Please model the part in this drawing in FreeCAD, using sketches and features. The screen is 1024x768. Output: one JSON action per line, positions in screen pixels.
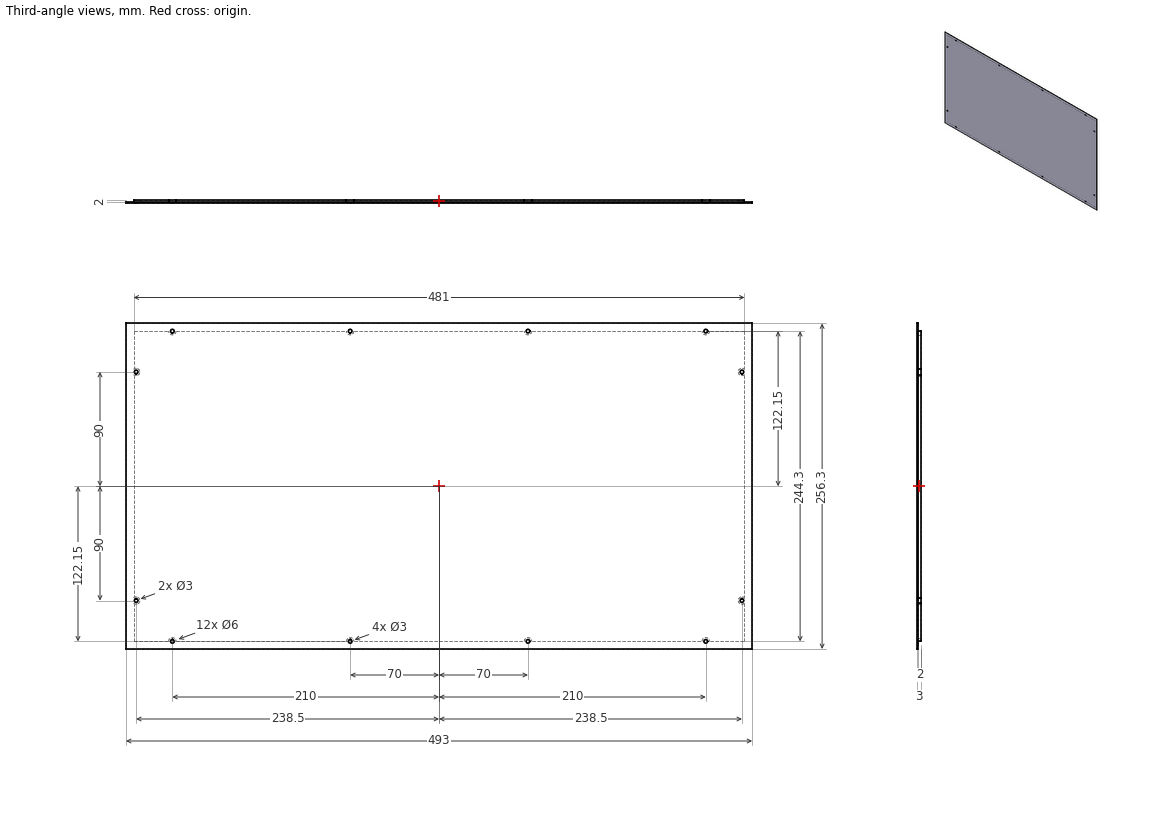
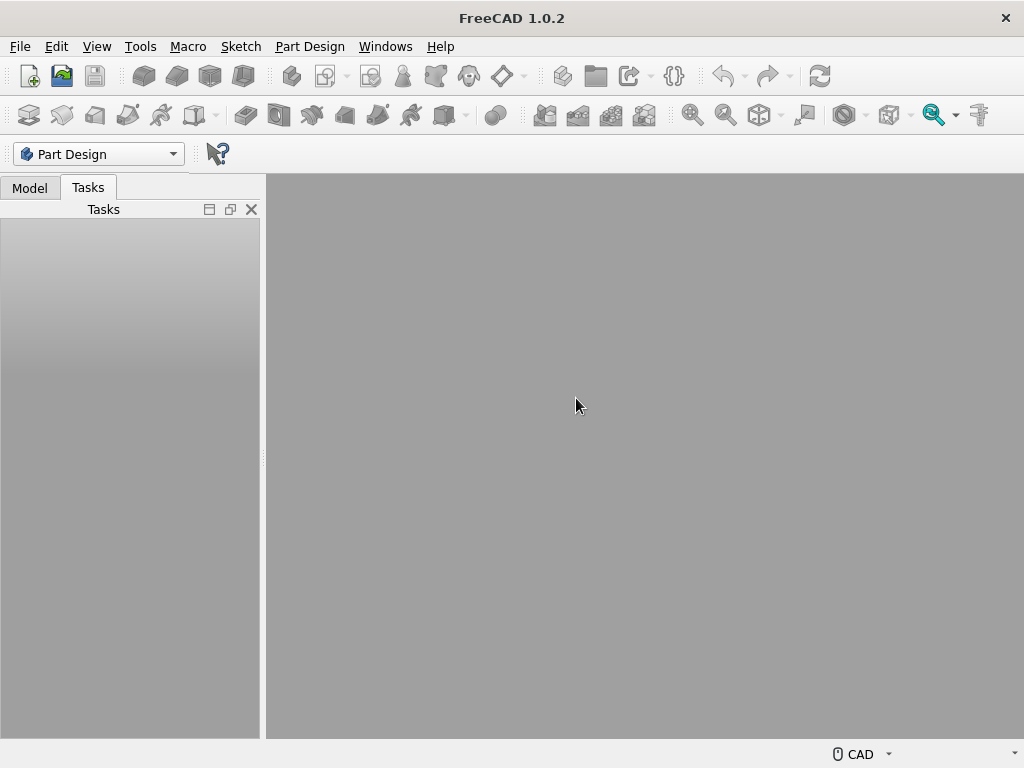
{"action": "left_click", "coordinate": [29, 76]}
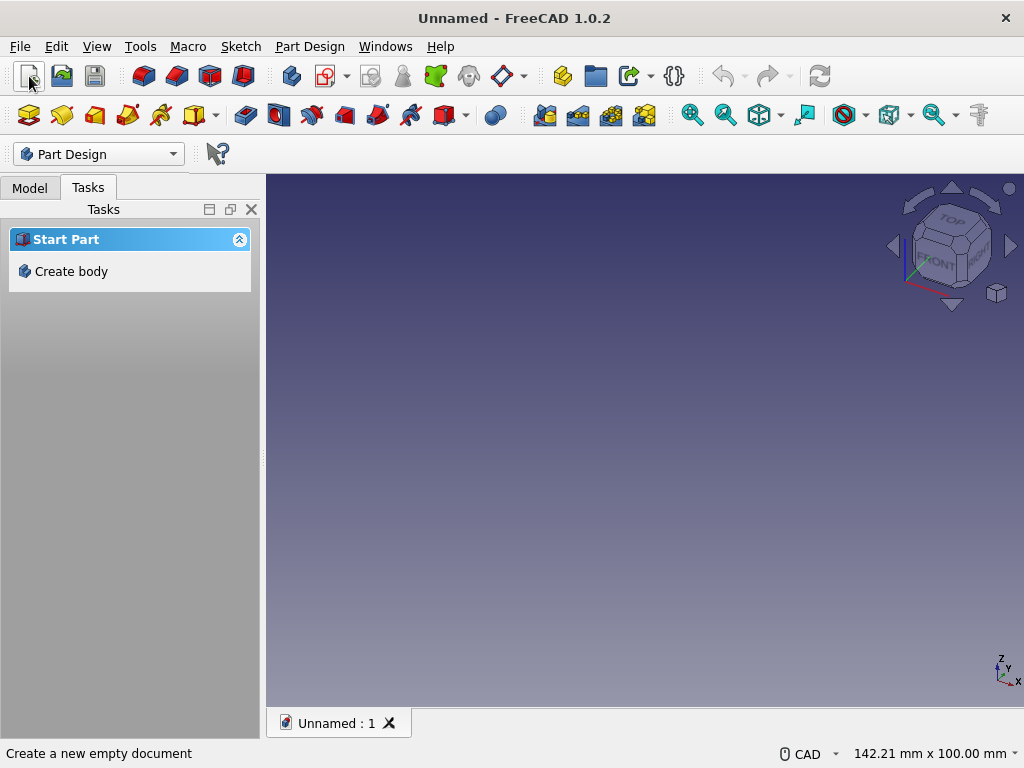
{"action": "left_click", "coordinate": [324, 76]}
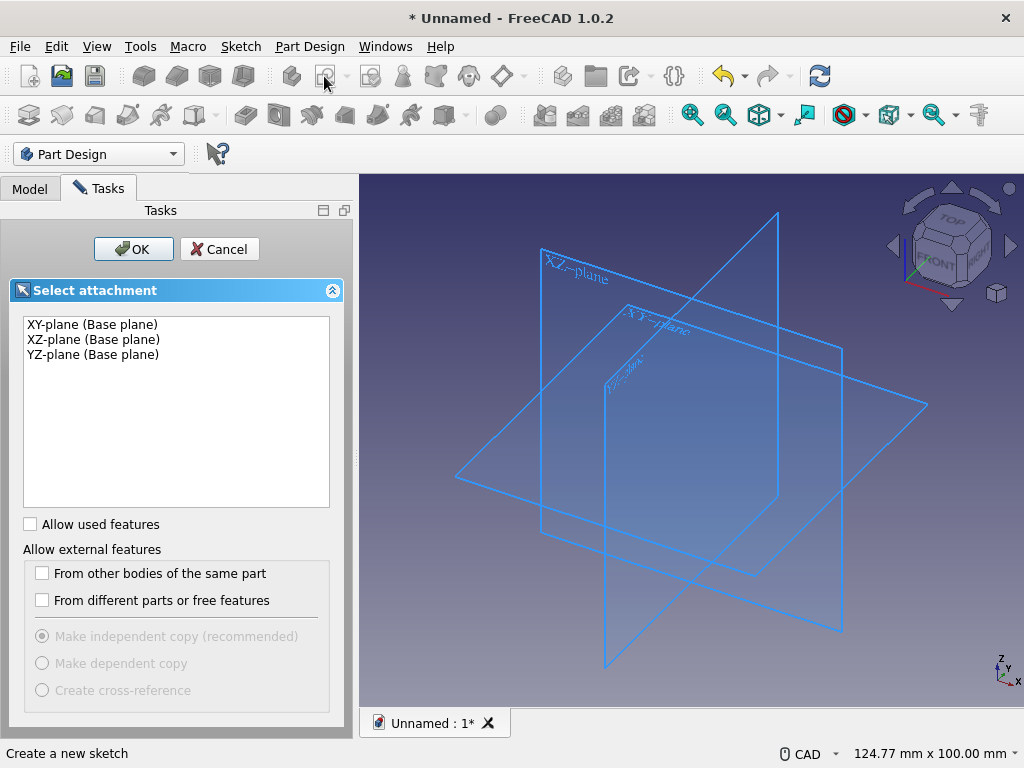
{"action": "left_click", "coordinate": [84, 340]}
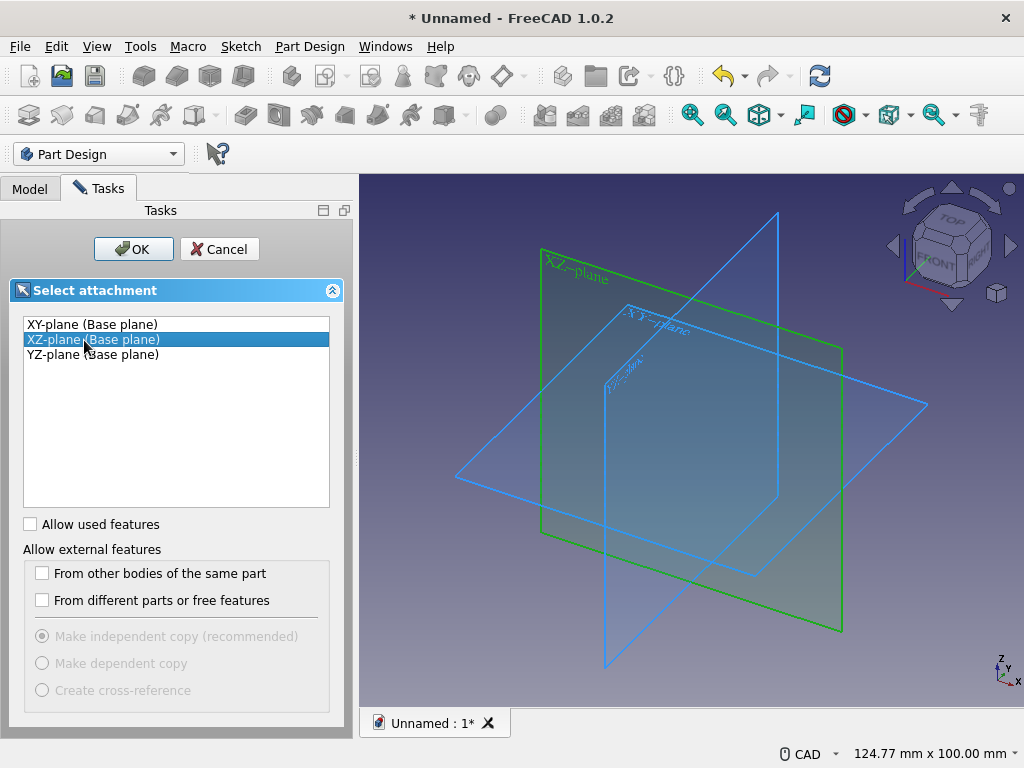
{"action": "left_click", "coordinate": [134, 249]}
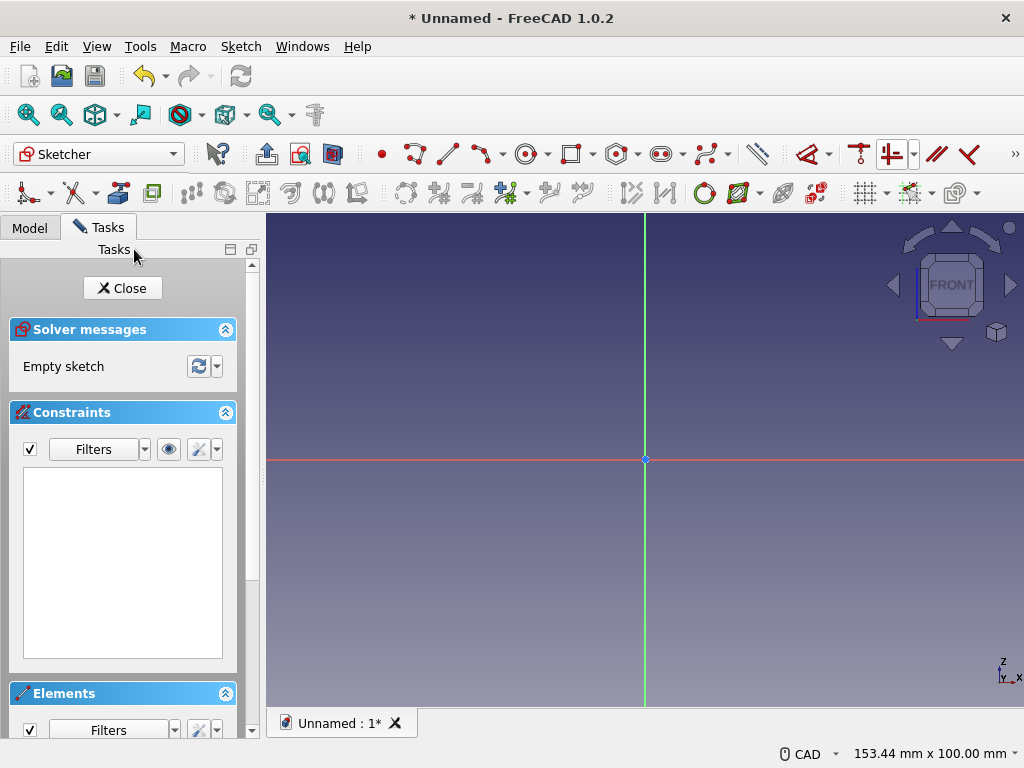
{"action": "scroll", "coordinate": [563, 460], "scroll_direction": "down", "scroll_amount": 9}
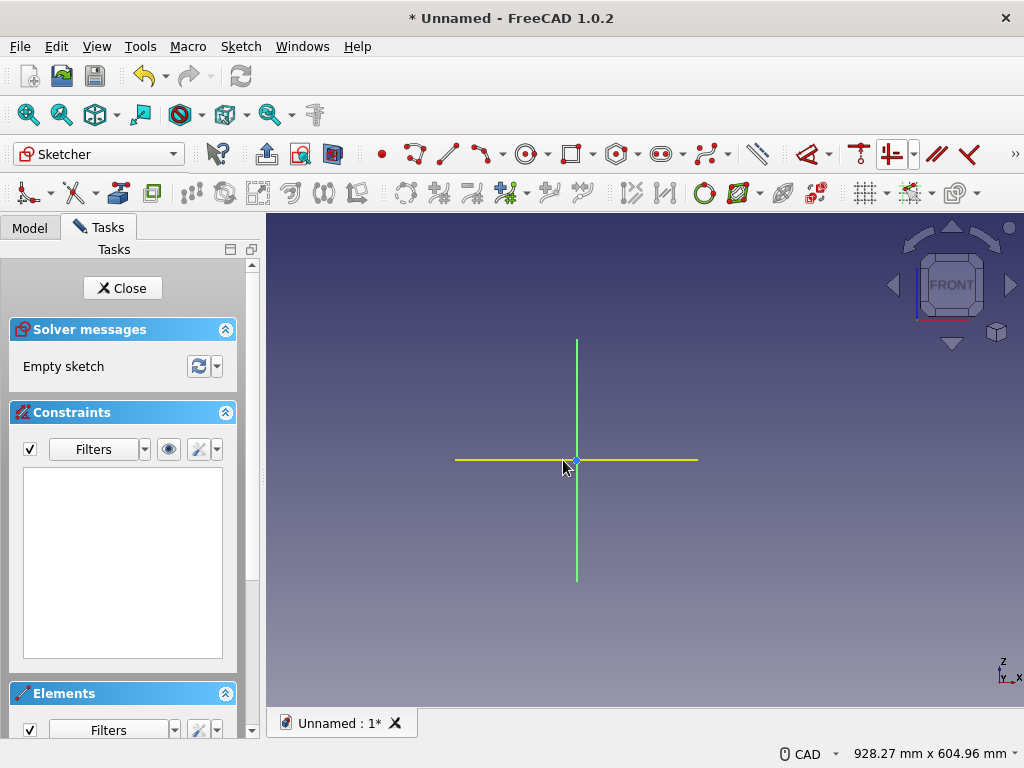
{"action": "left_click", "coordinate": [592, 154]}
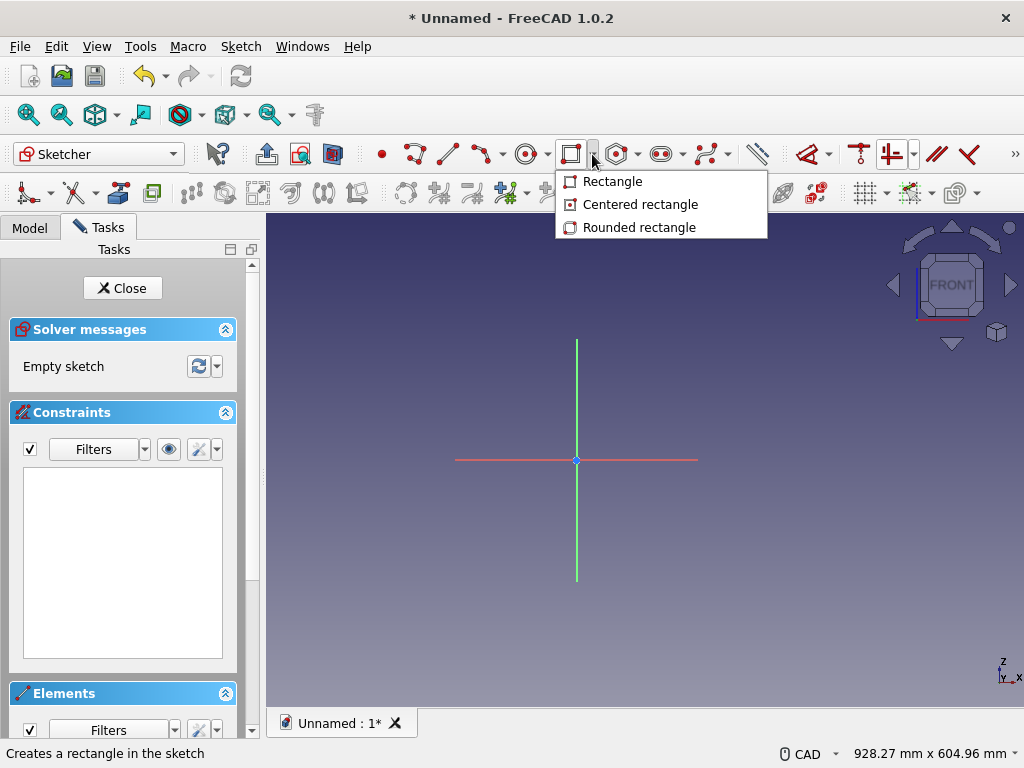
{"action": "left_click", "coordinate": [662, 204]}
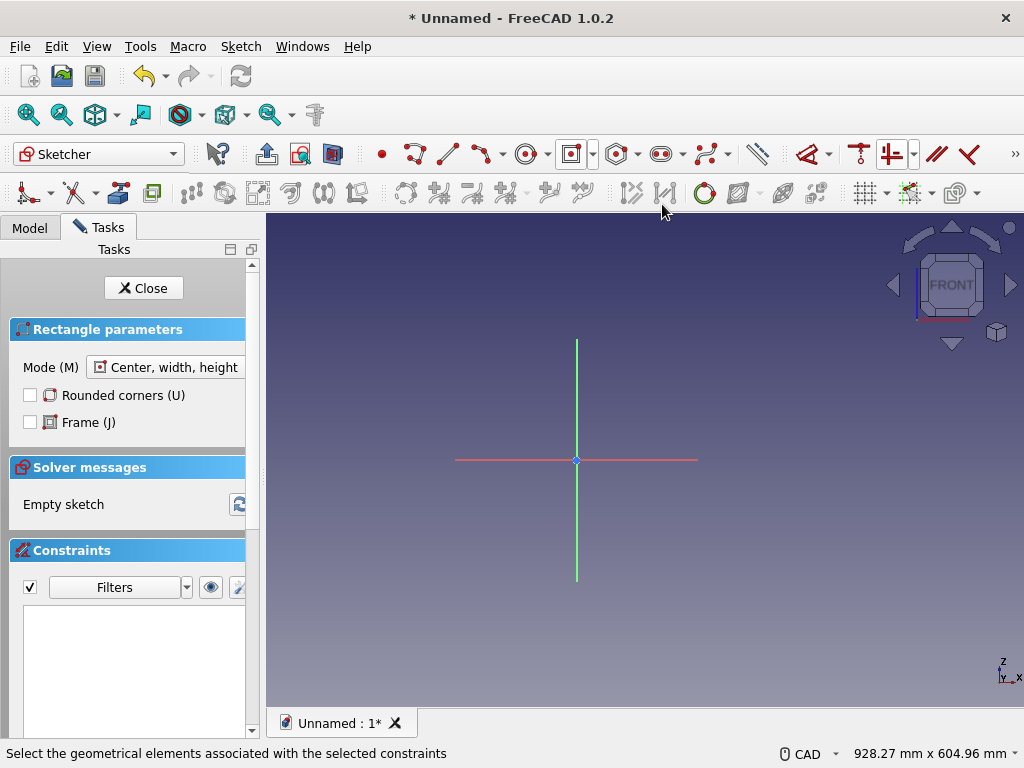
{"action": "left_click", "coordinate": [577, 460]}
{"action": "left_click", "coordinate": [778, 356]}
{"action": "key", "text": "Escape"}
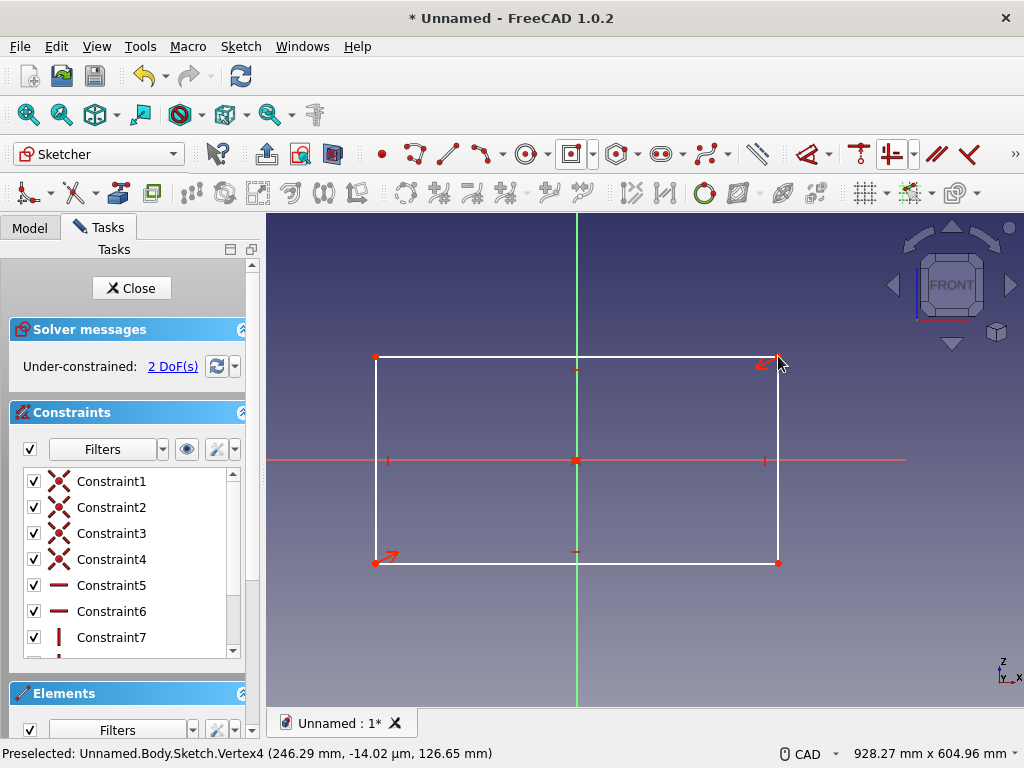
{"action": "left_click", "coordinate": [806, 154]}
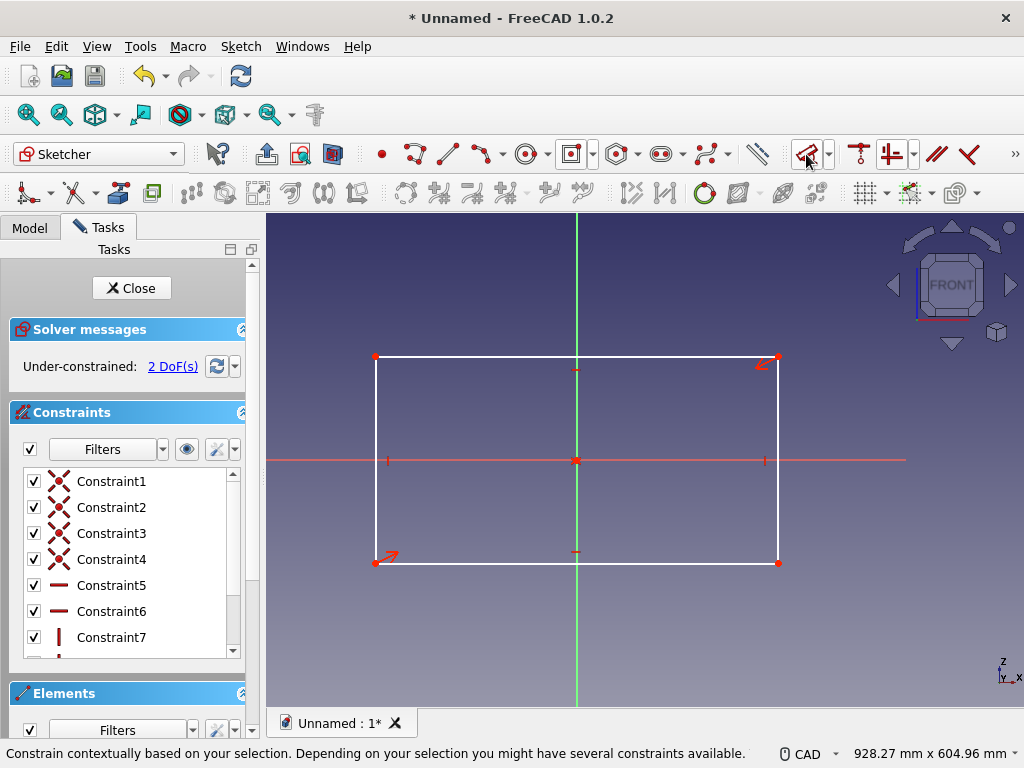
{"action": "left_click", "coordinate": [496, 564]}
{"action": "left_click", "coordinate": [484, 598]}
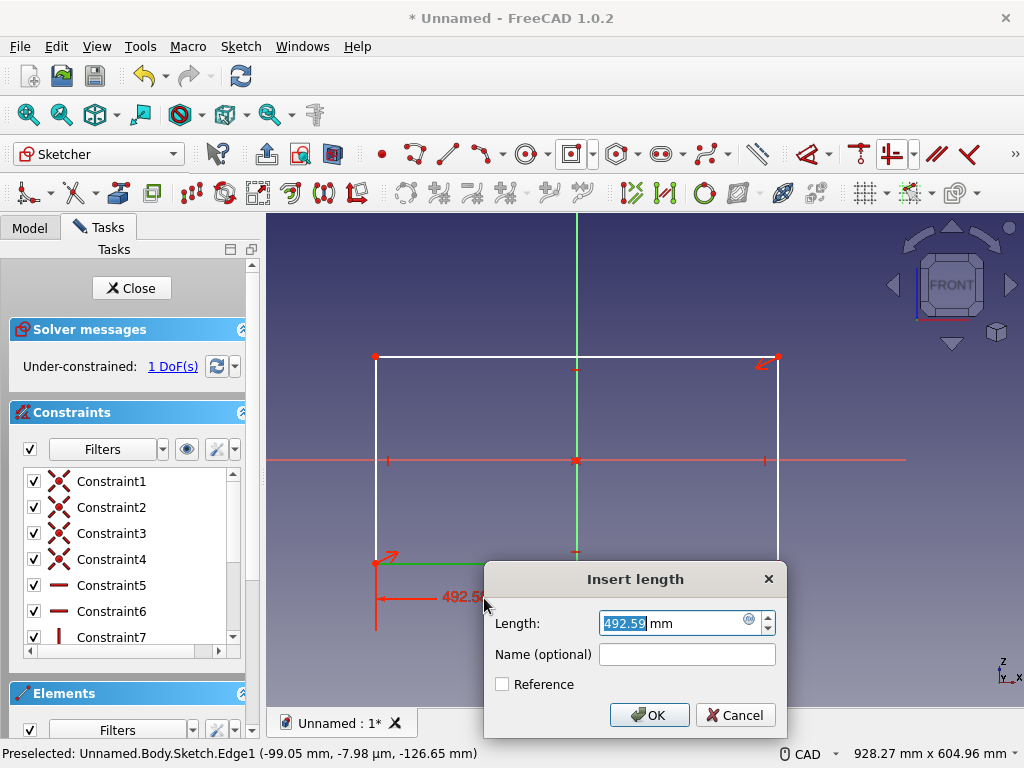
{"action": "type", "text": "493"}
{"action": "key", "text": "Return"}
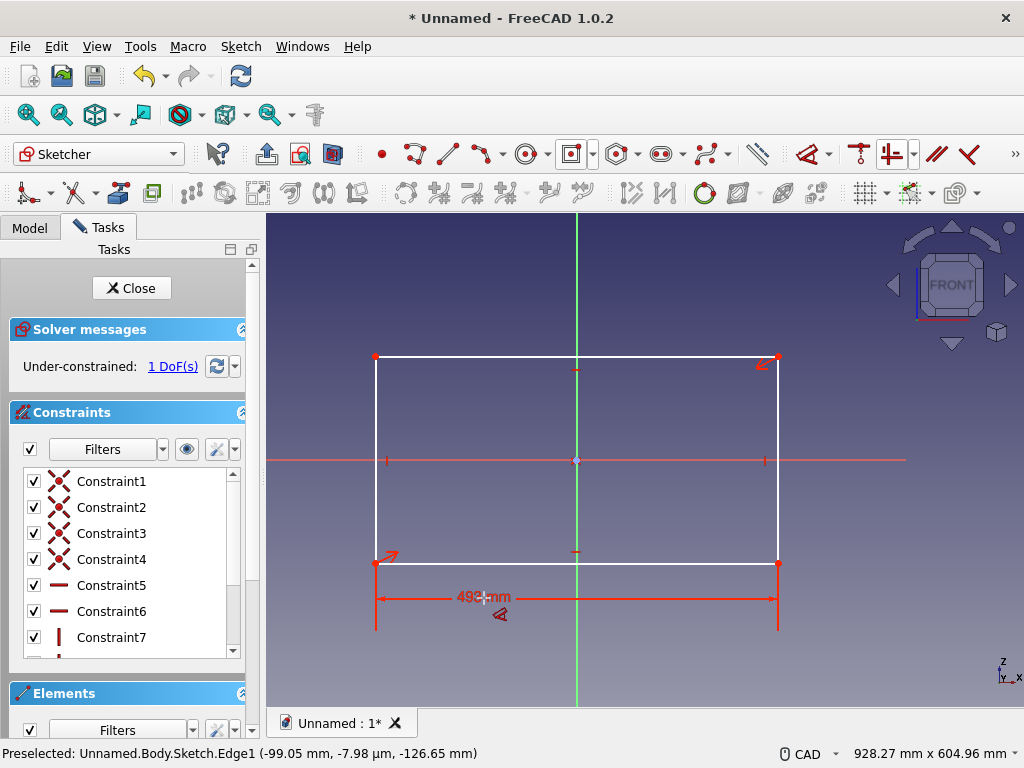
{"action": "left_click", "coordinate": [778, 502]}
{"action": "left_click", "coordinate": [812, 413]}